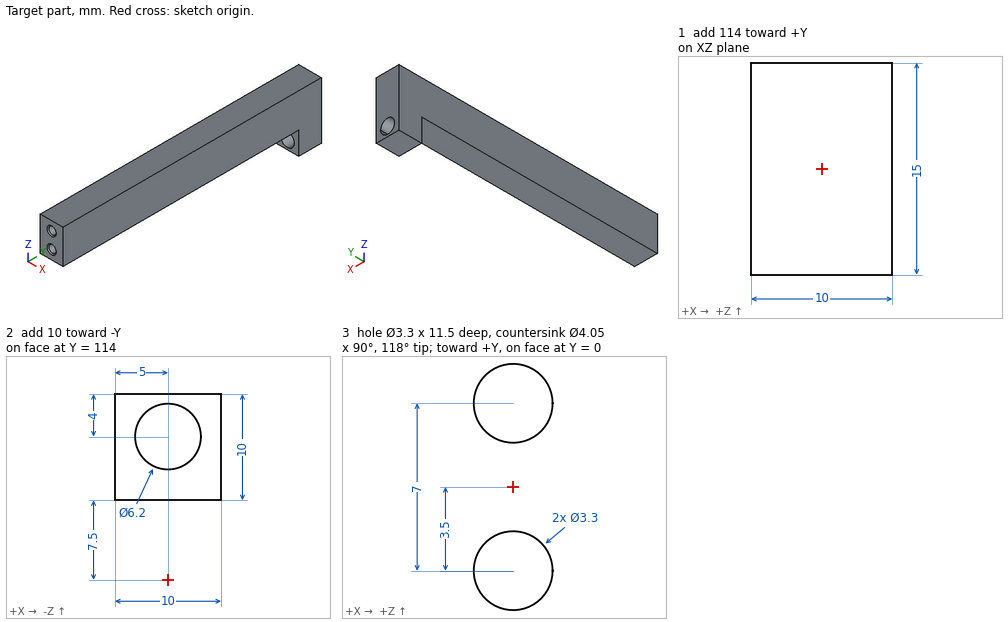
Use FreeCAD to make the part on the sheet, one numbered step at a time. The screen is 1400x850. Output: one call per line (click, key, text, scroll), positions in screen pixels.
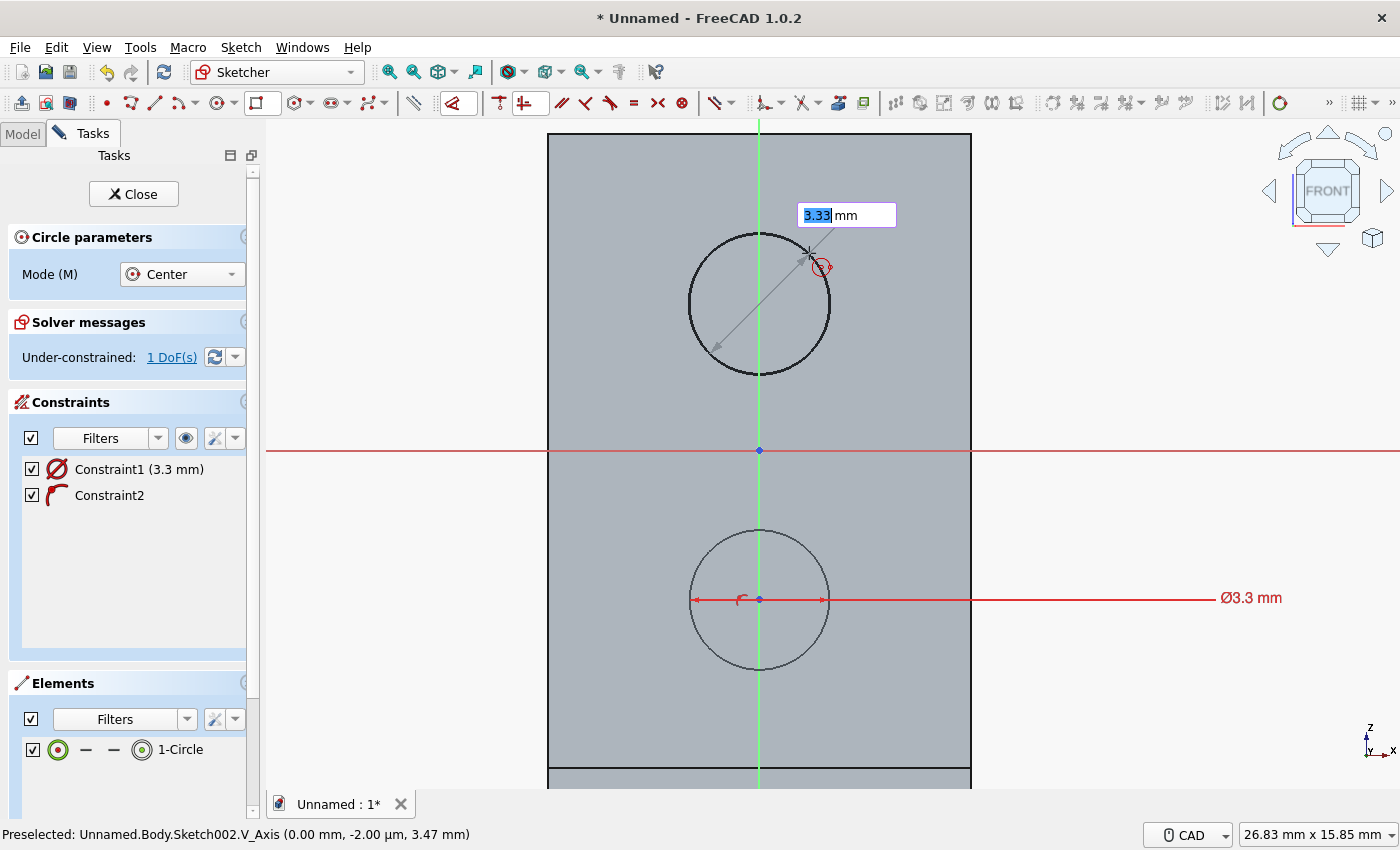
text(3.3)
key(Return)
key(Escape)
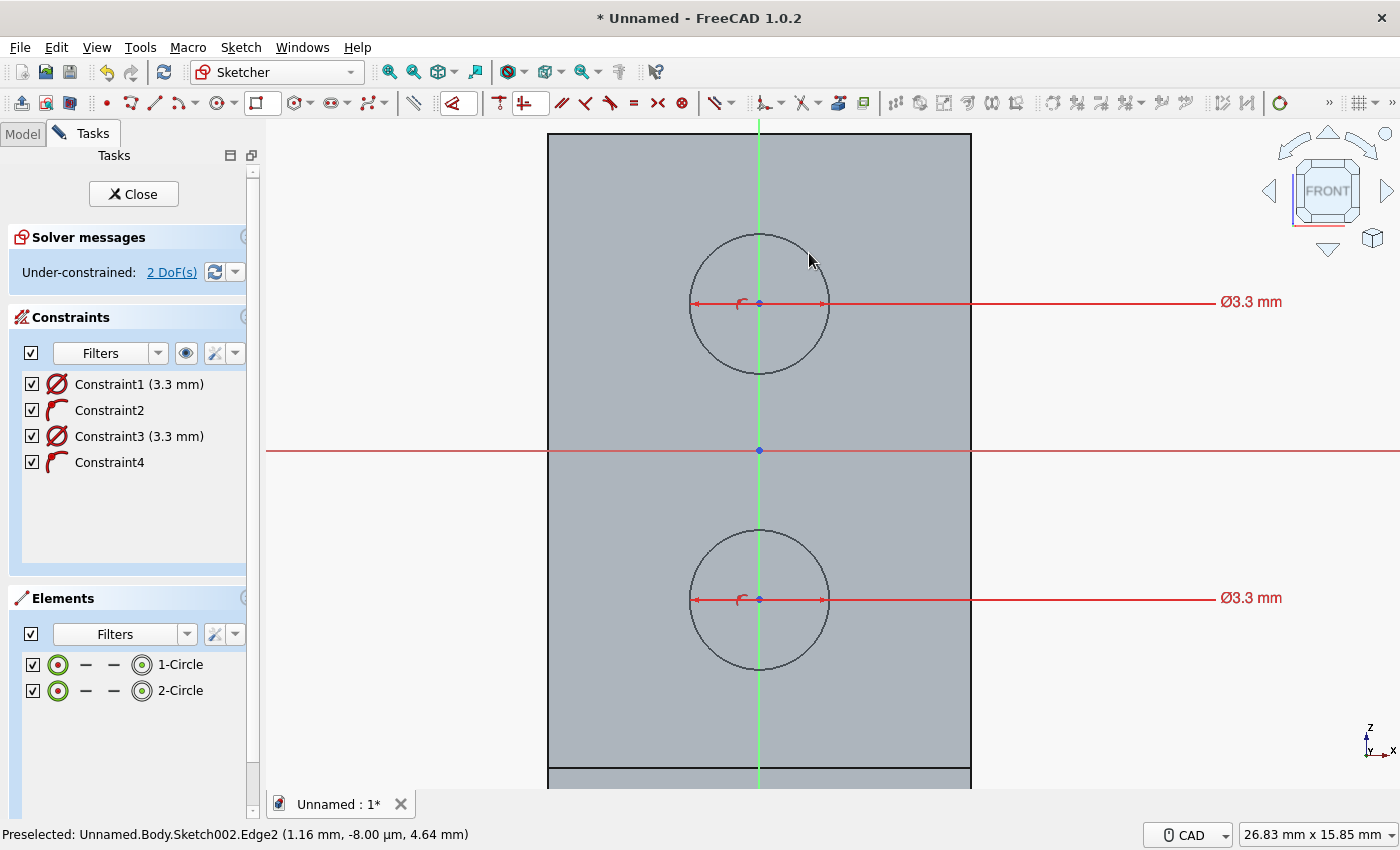
click(759, 600)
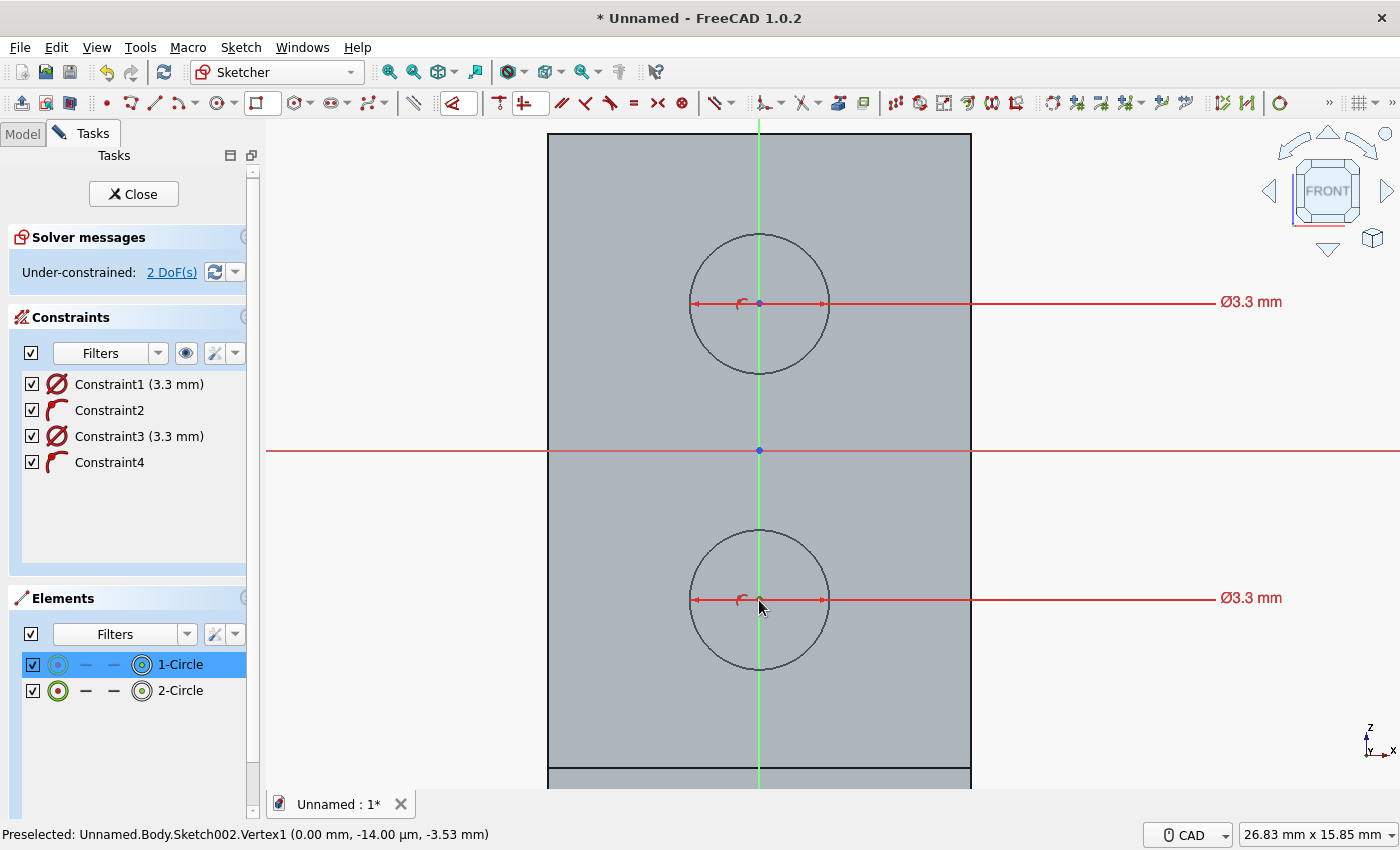
click(759, 304)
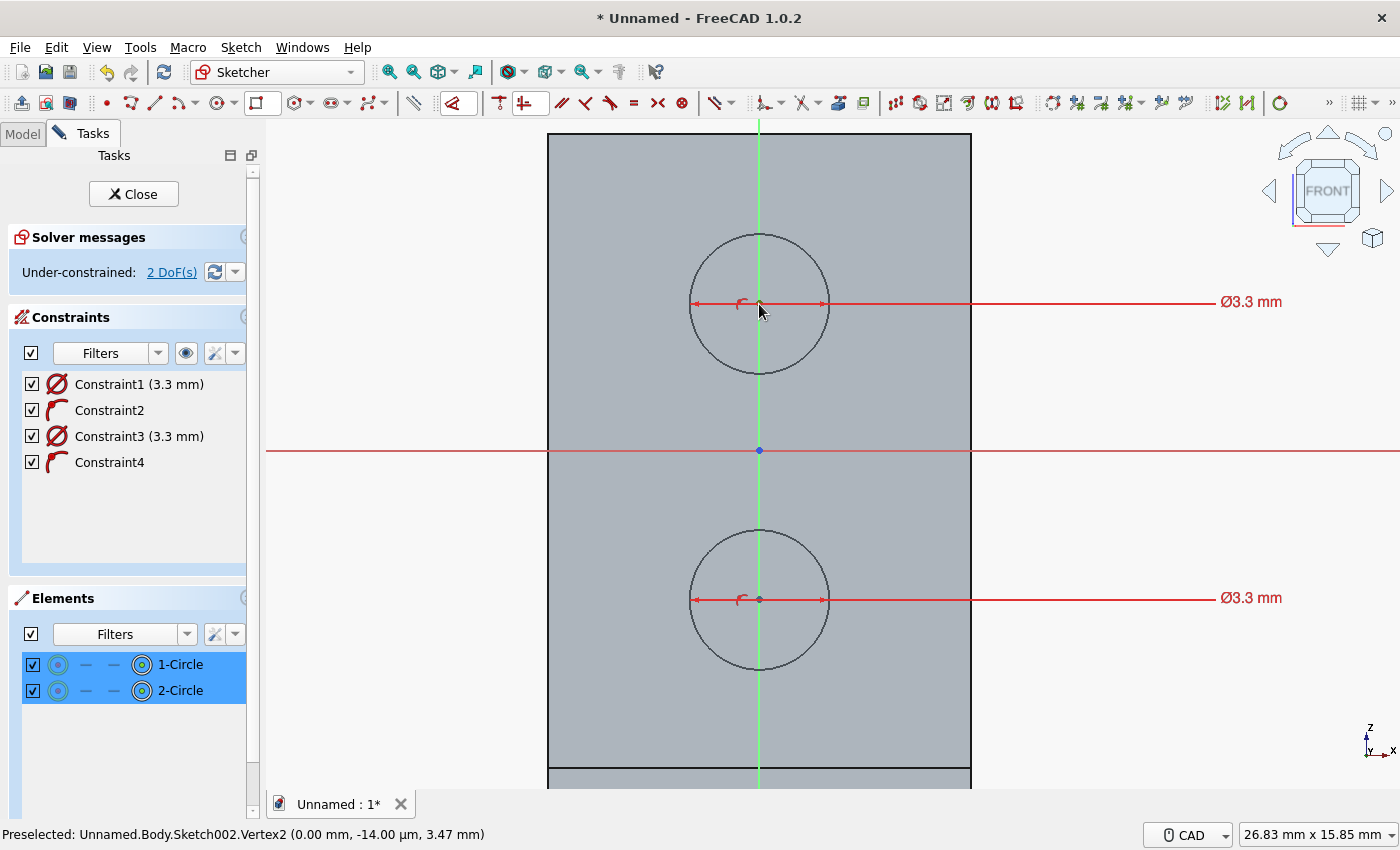
key(i)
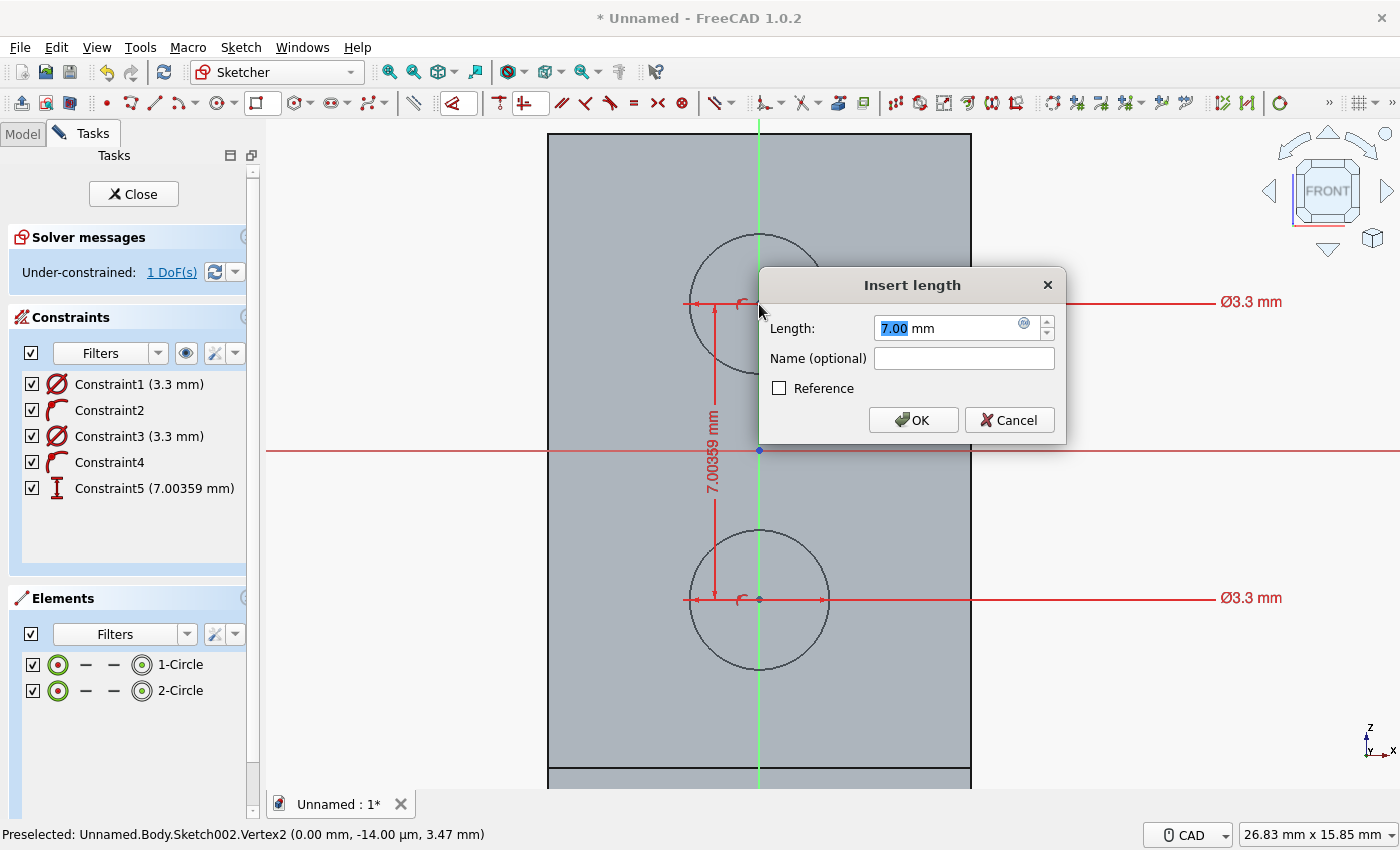
text(7)
key(Return)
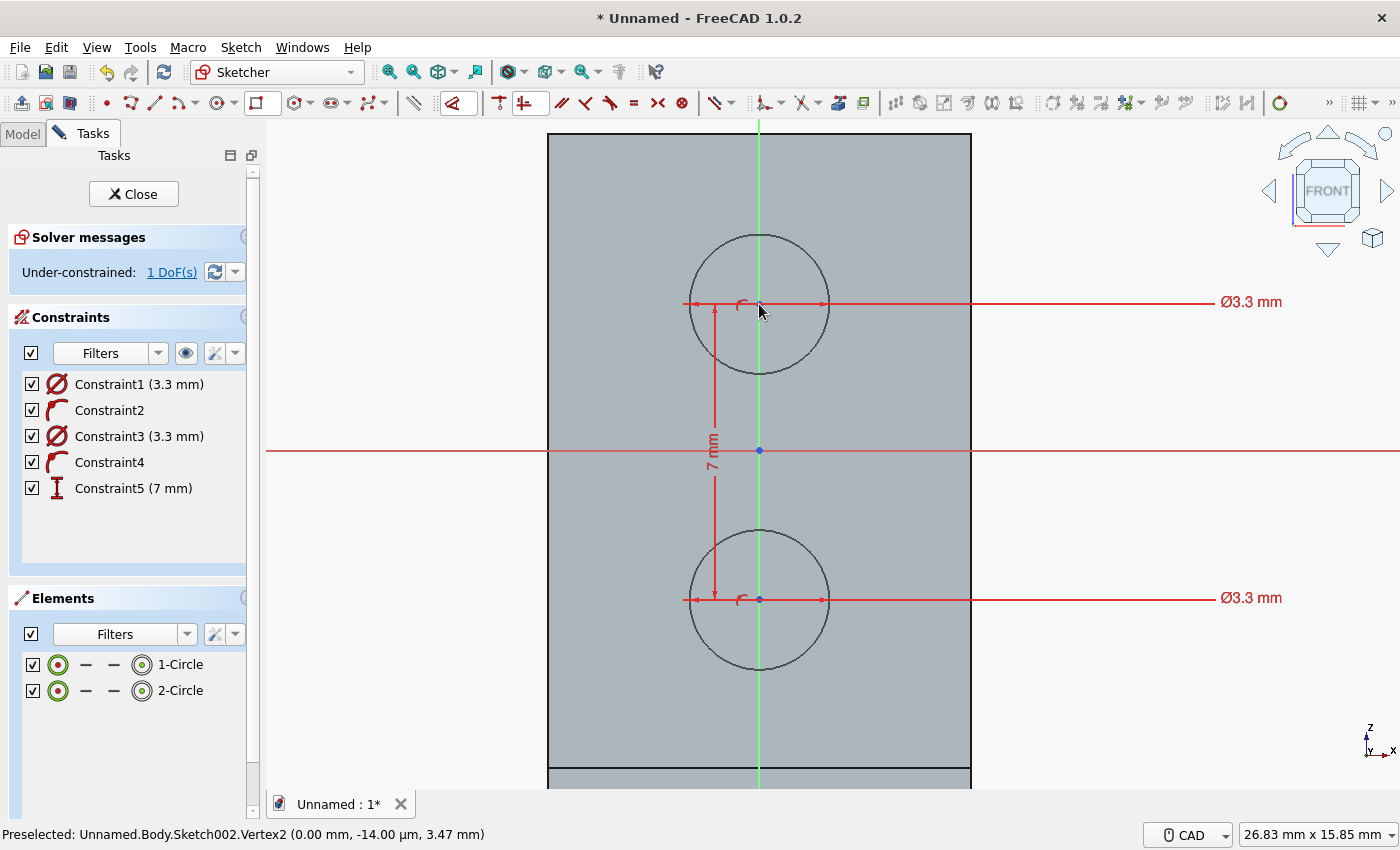
click(759, 600)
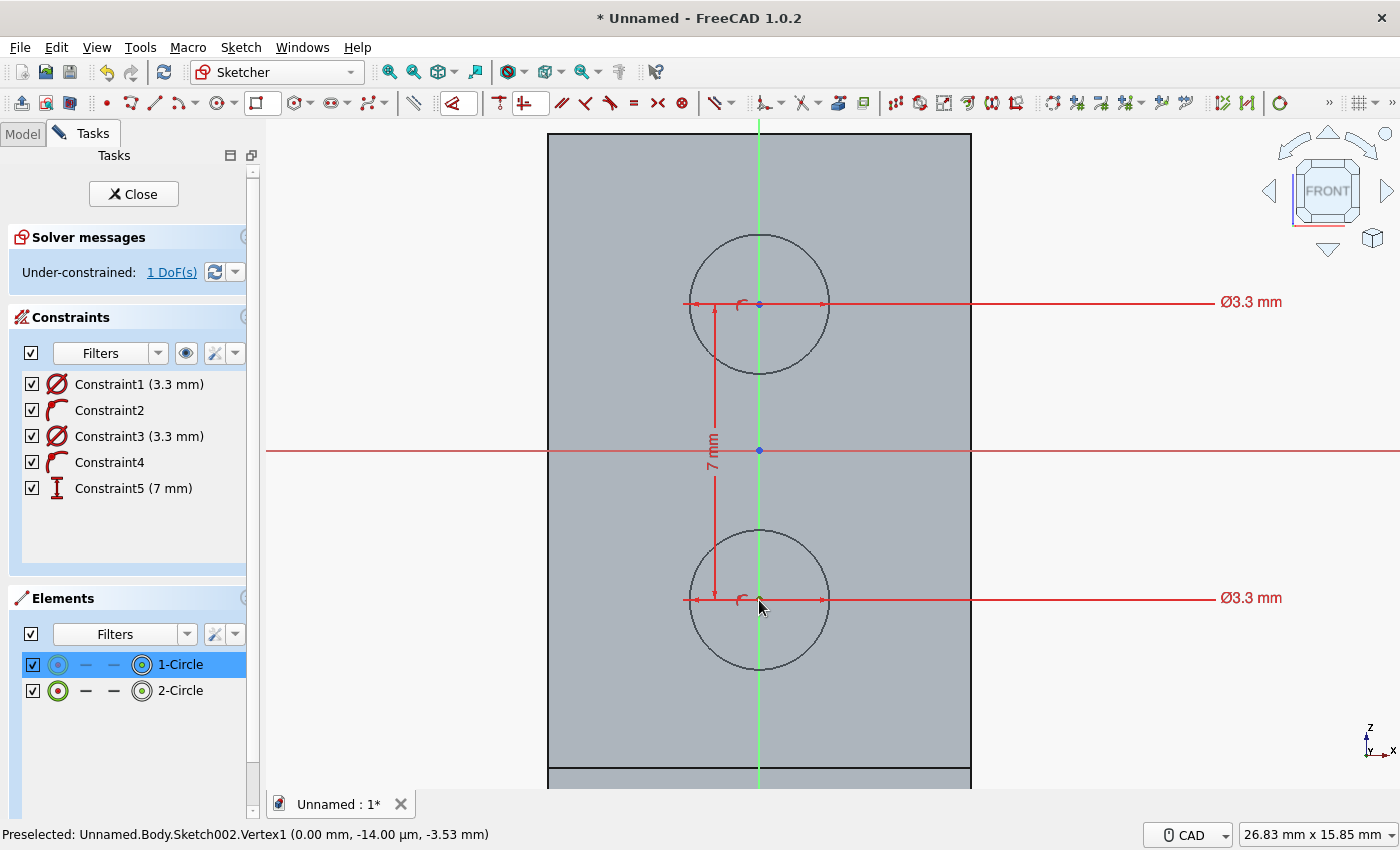
key(i)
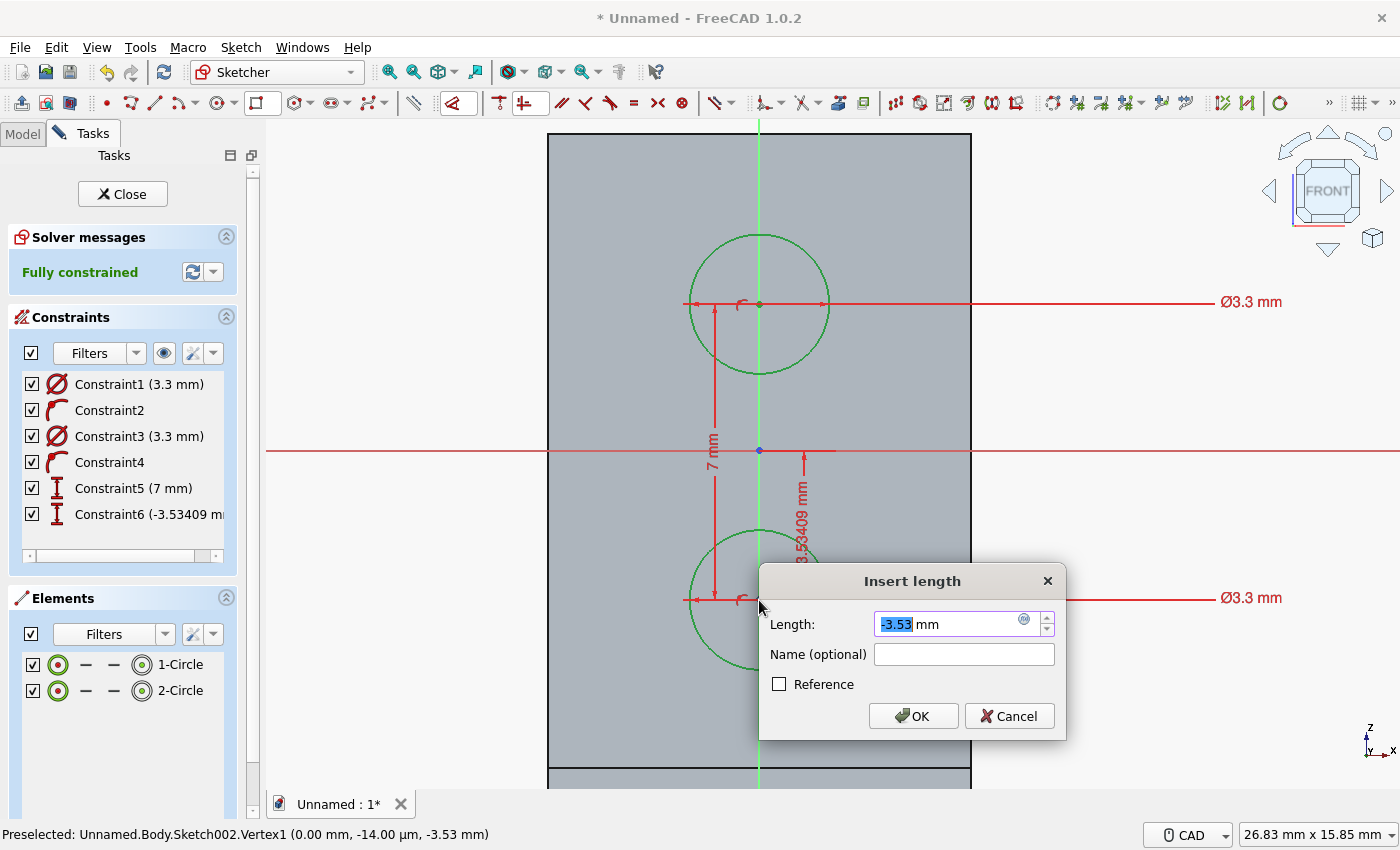
text(-3.5)
key(Return)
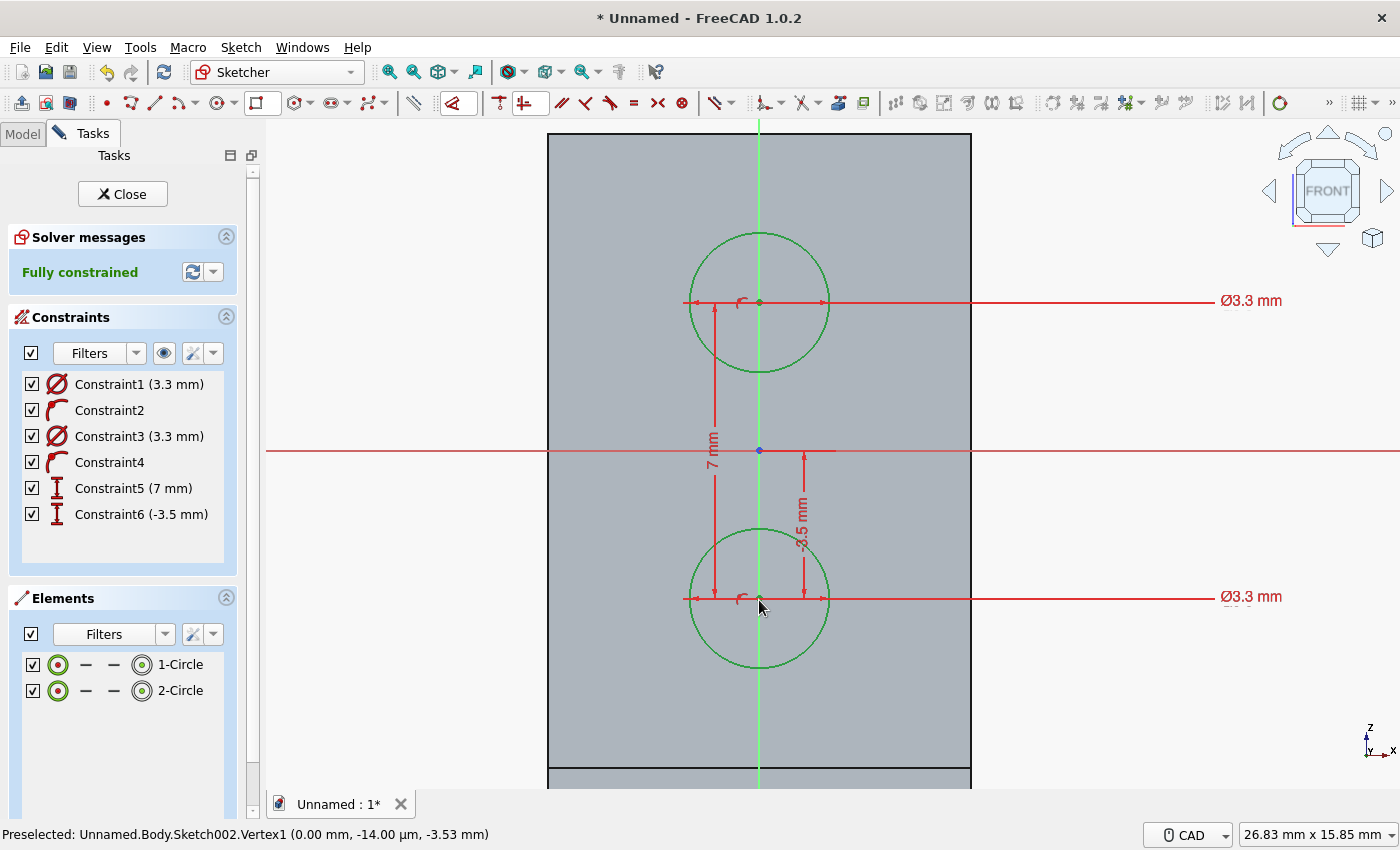
click(123, 194)